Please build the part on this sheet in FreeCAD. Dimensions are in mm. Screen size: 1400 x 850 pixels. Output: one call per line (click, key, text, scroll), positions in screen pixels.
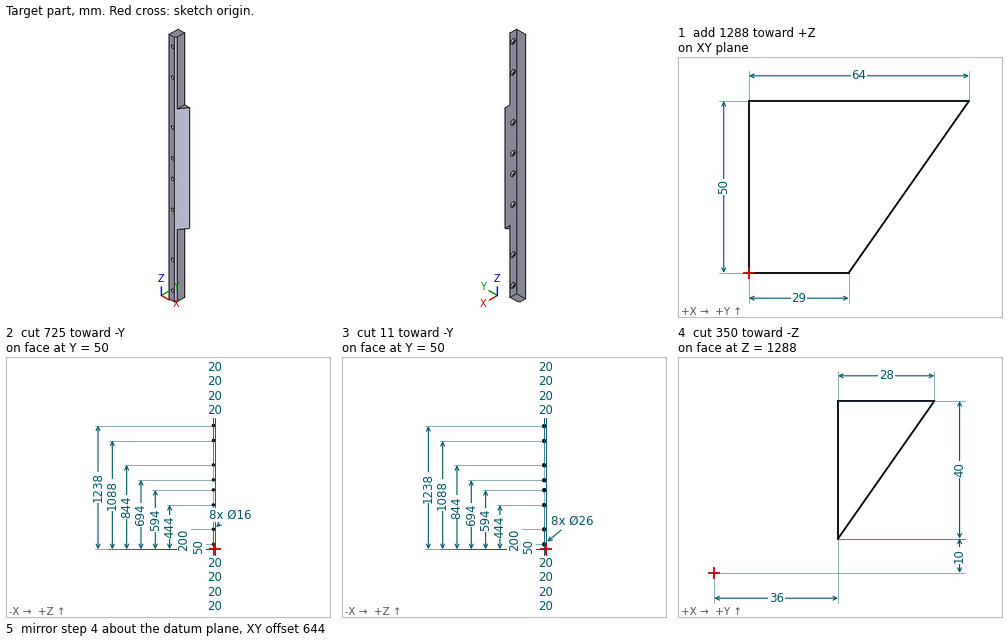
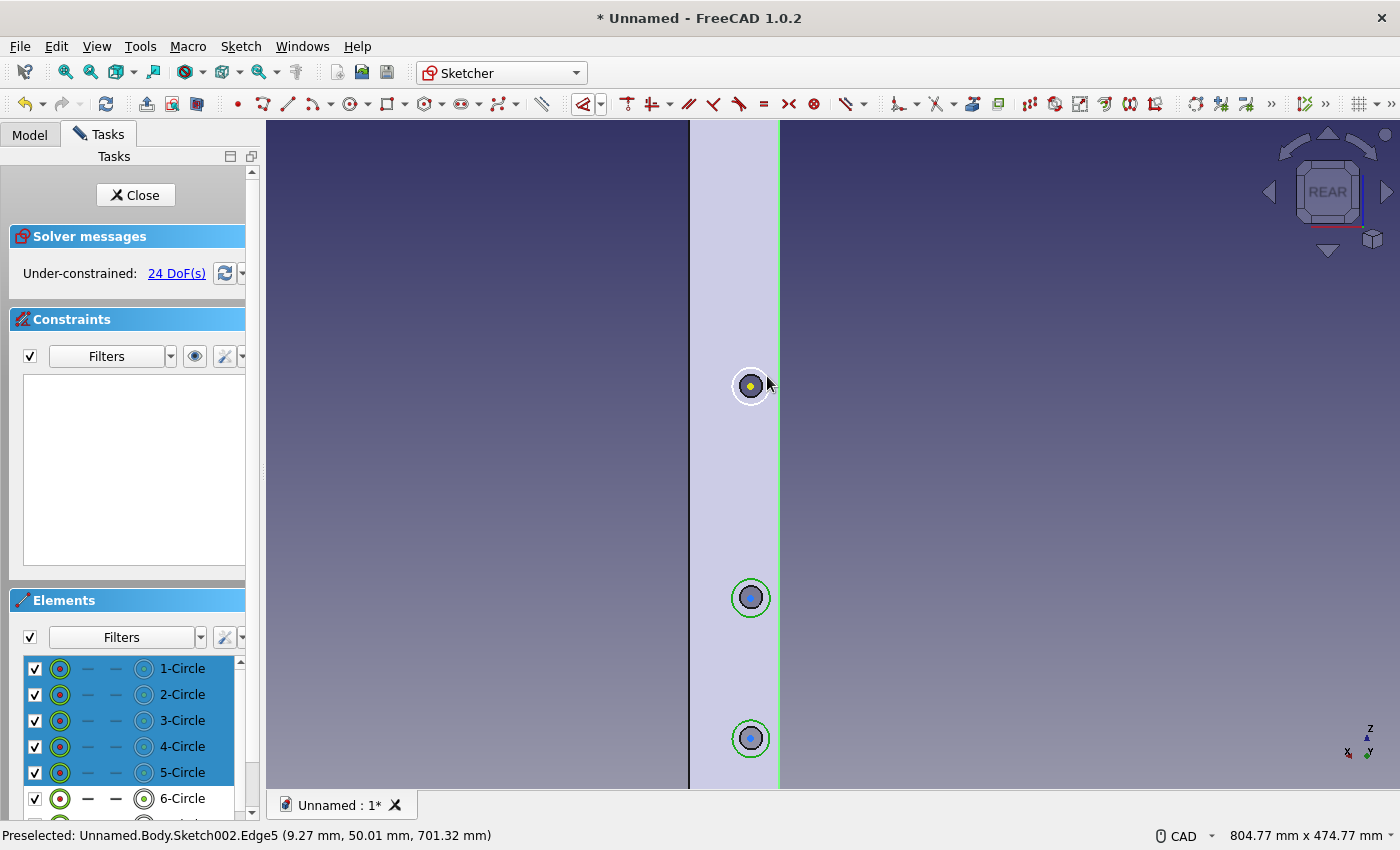
click(764, 373)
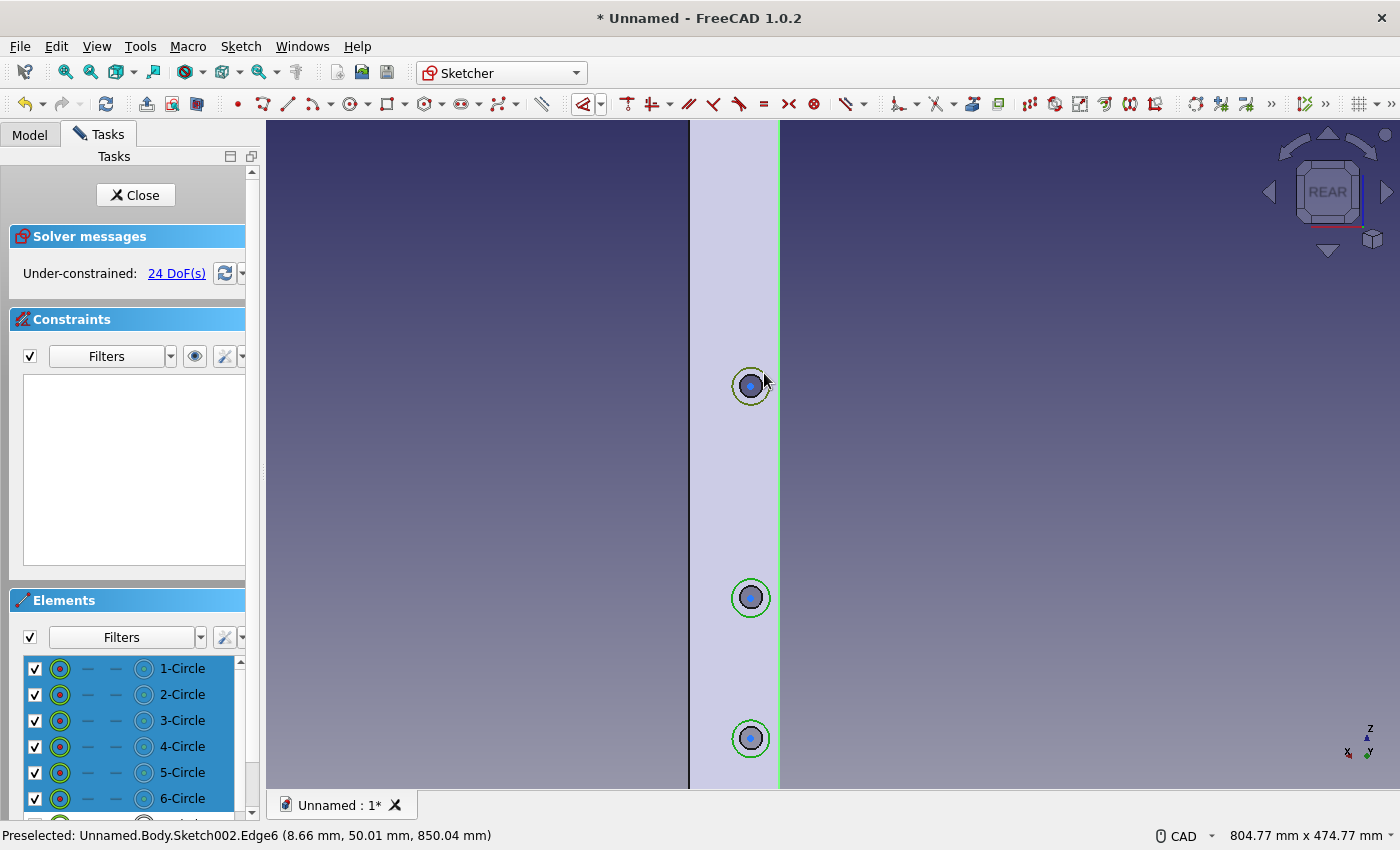
scroll(767, 376, down, 7)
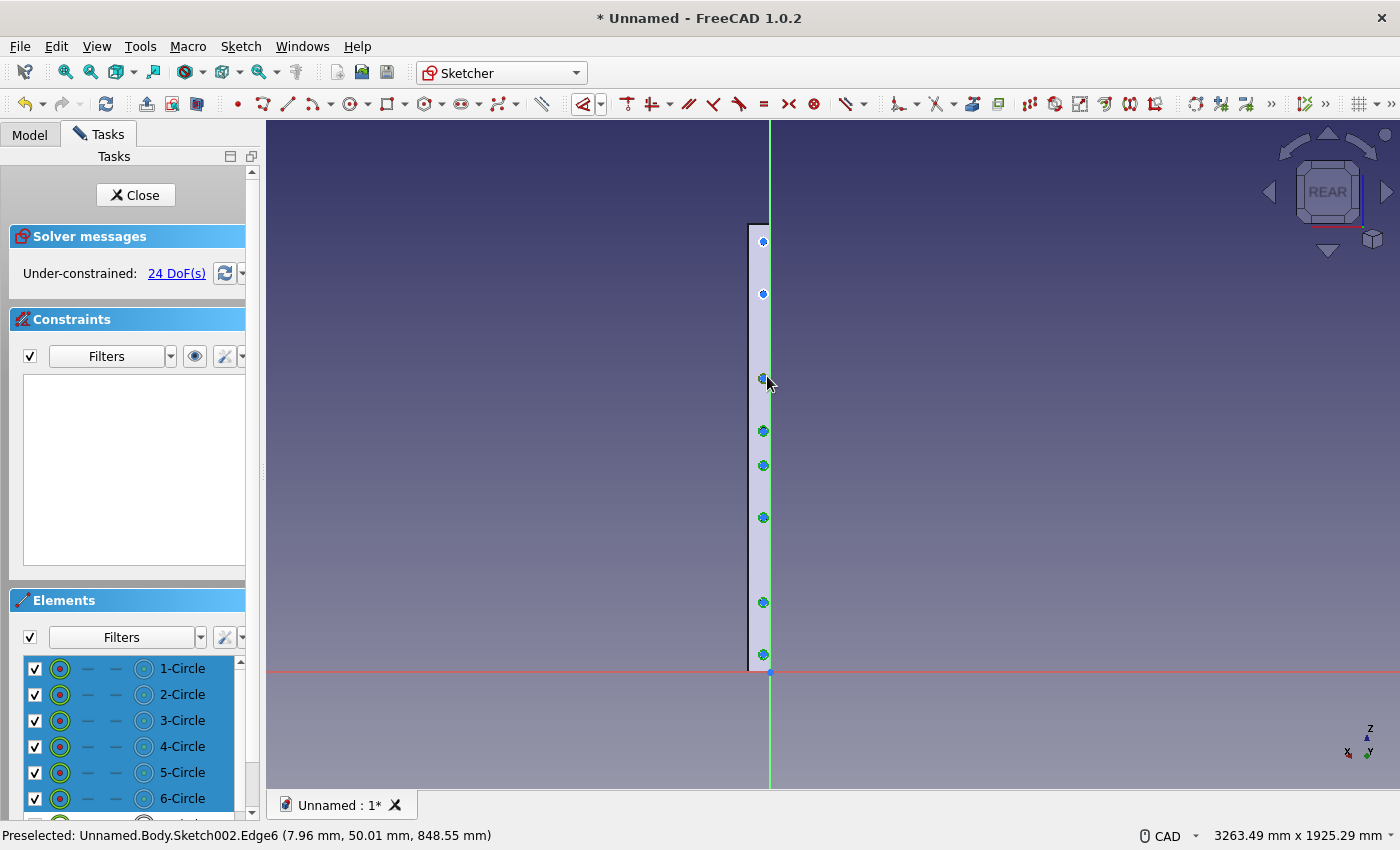
scroll(767, 291, up, 7)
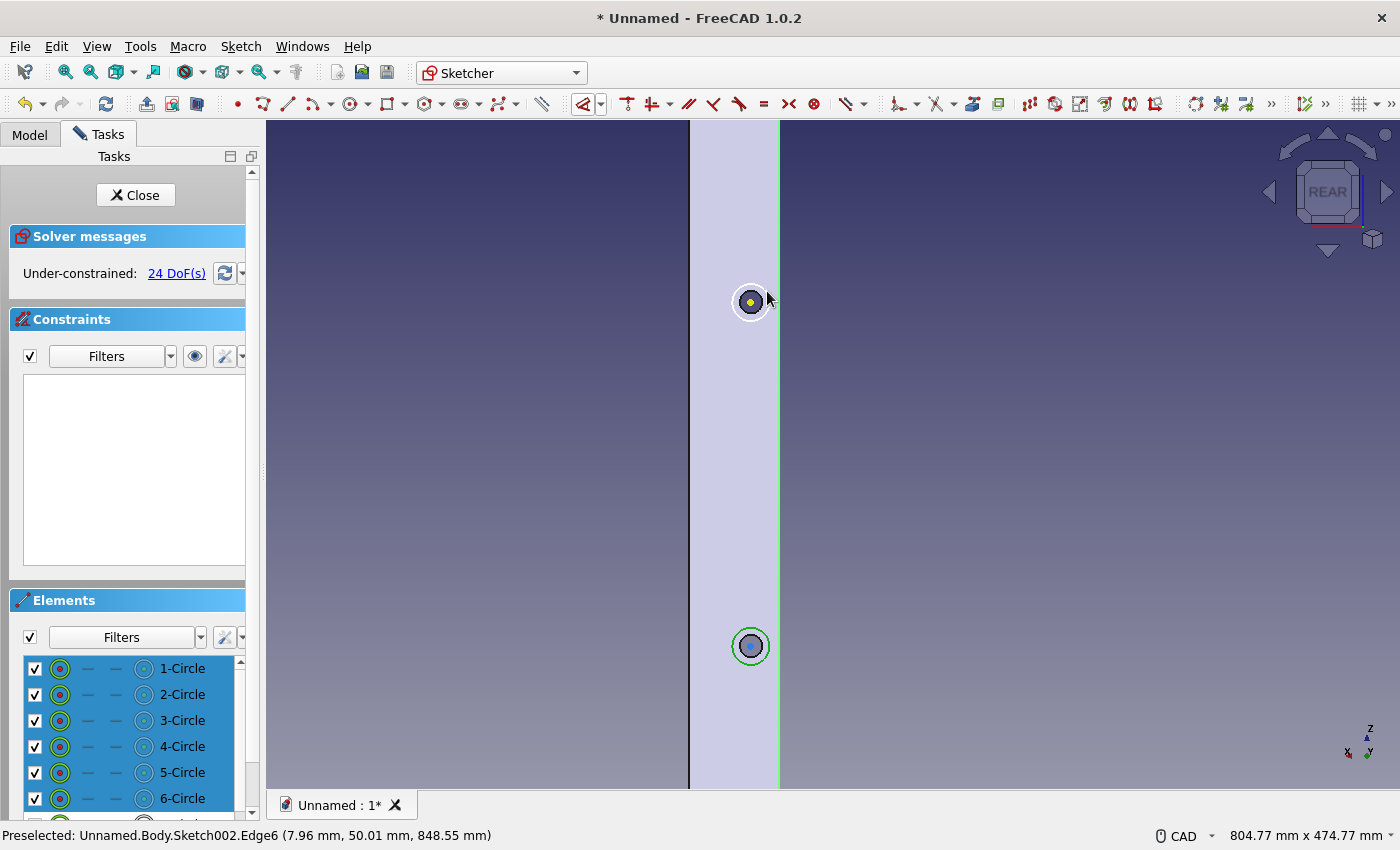
click(764, 289)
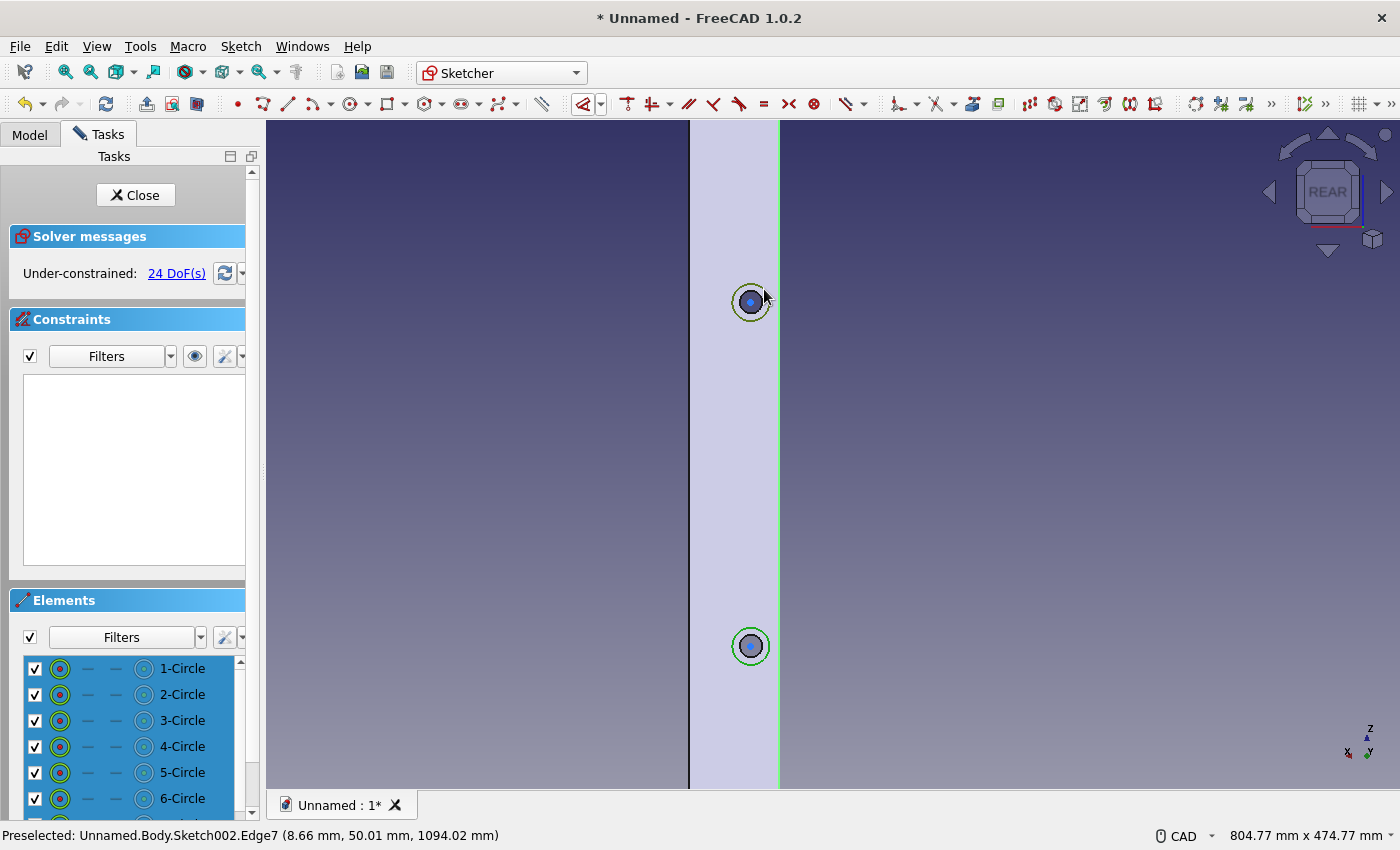
scroll(767, 291, down, 7)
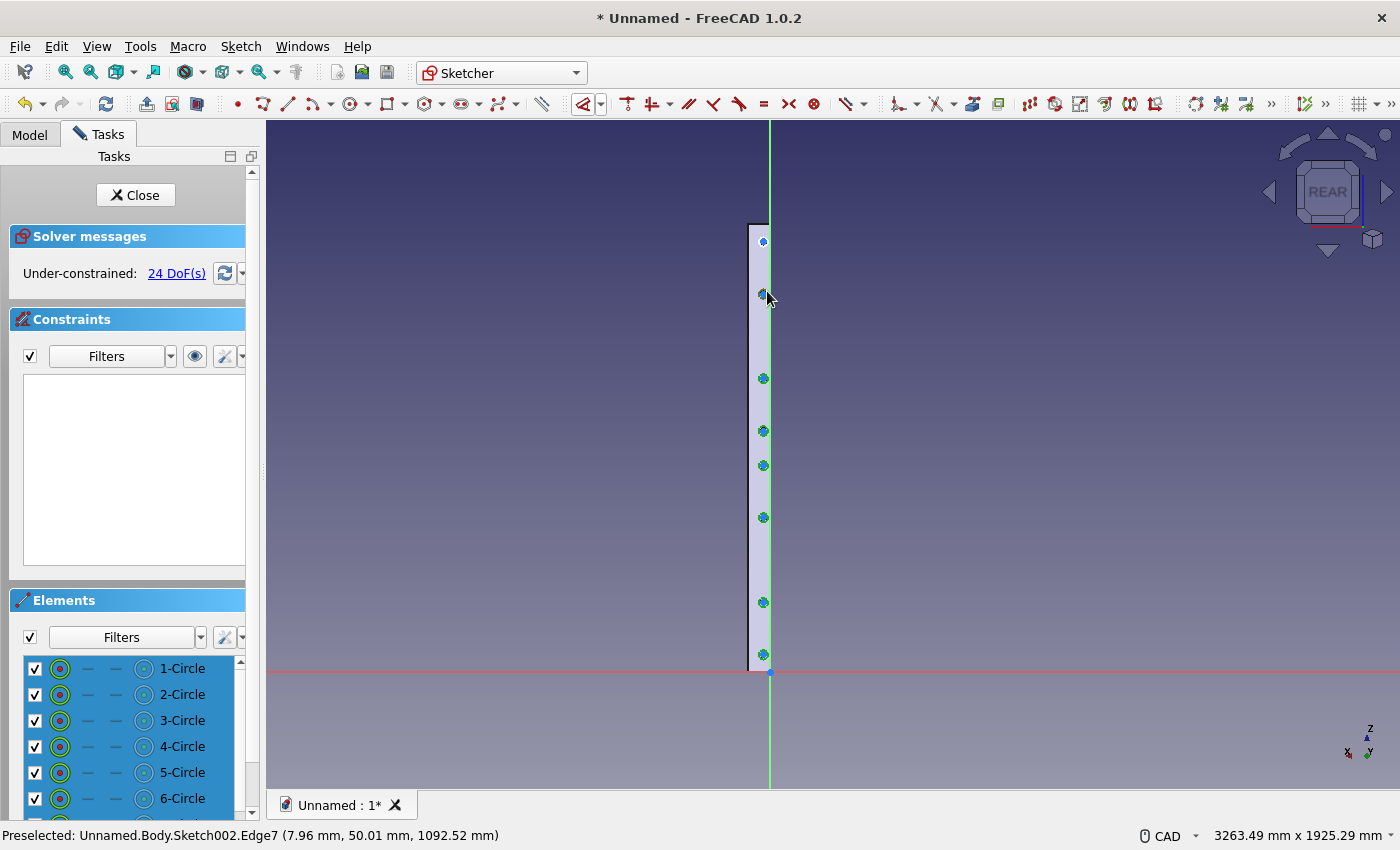
scroll(767, 239, up, 7)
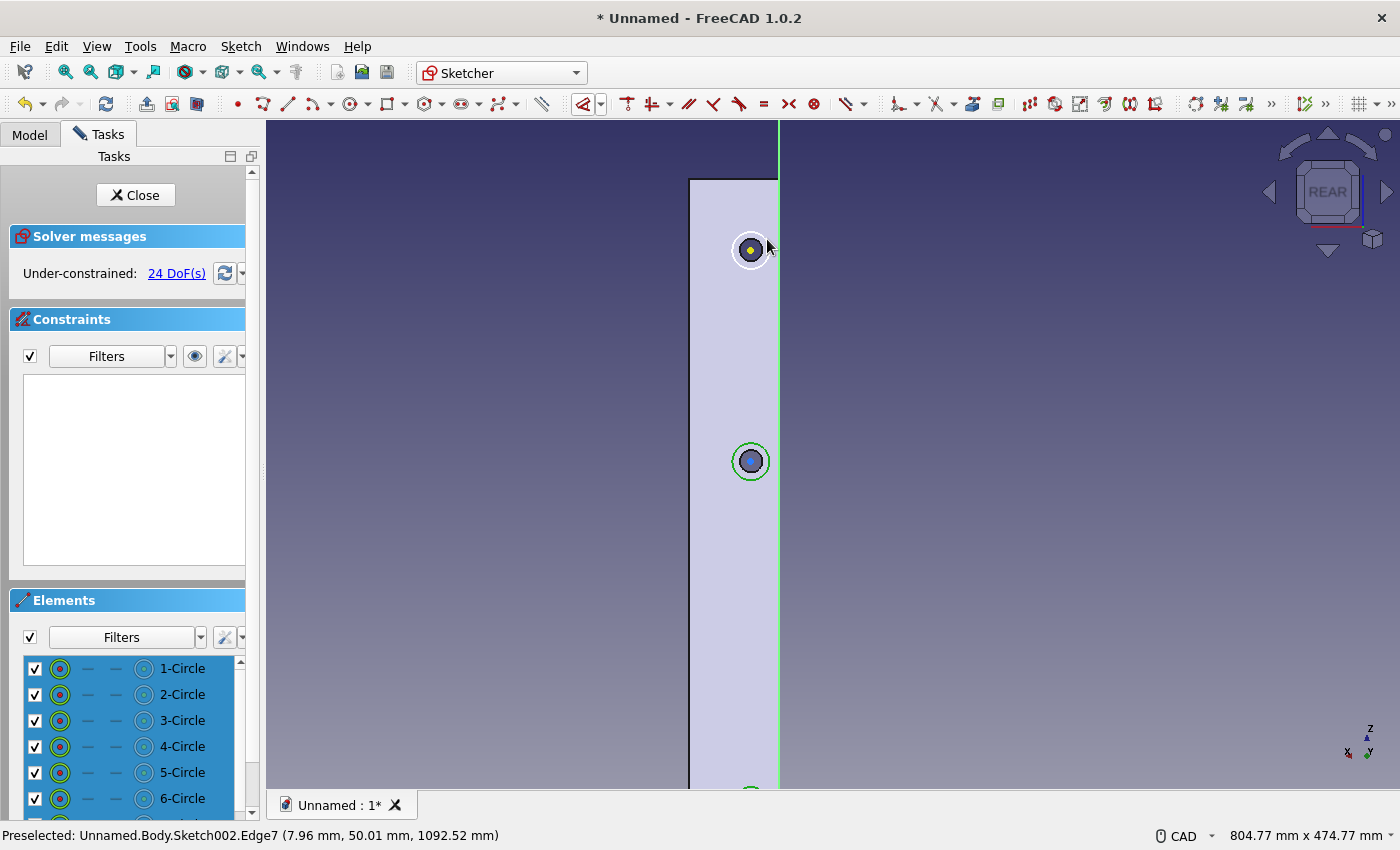
click(764, 237)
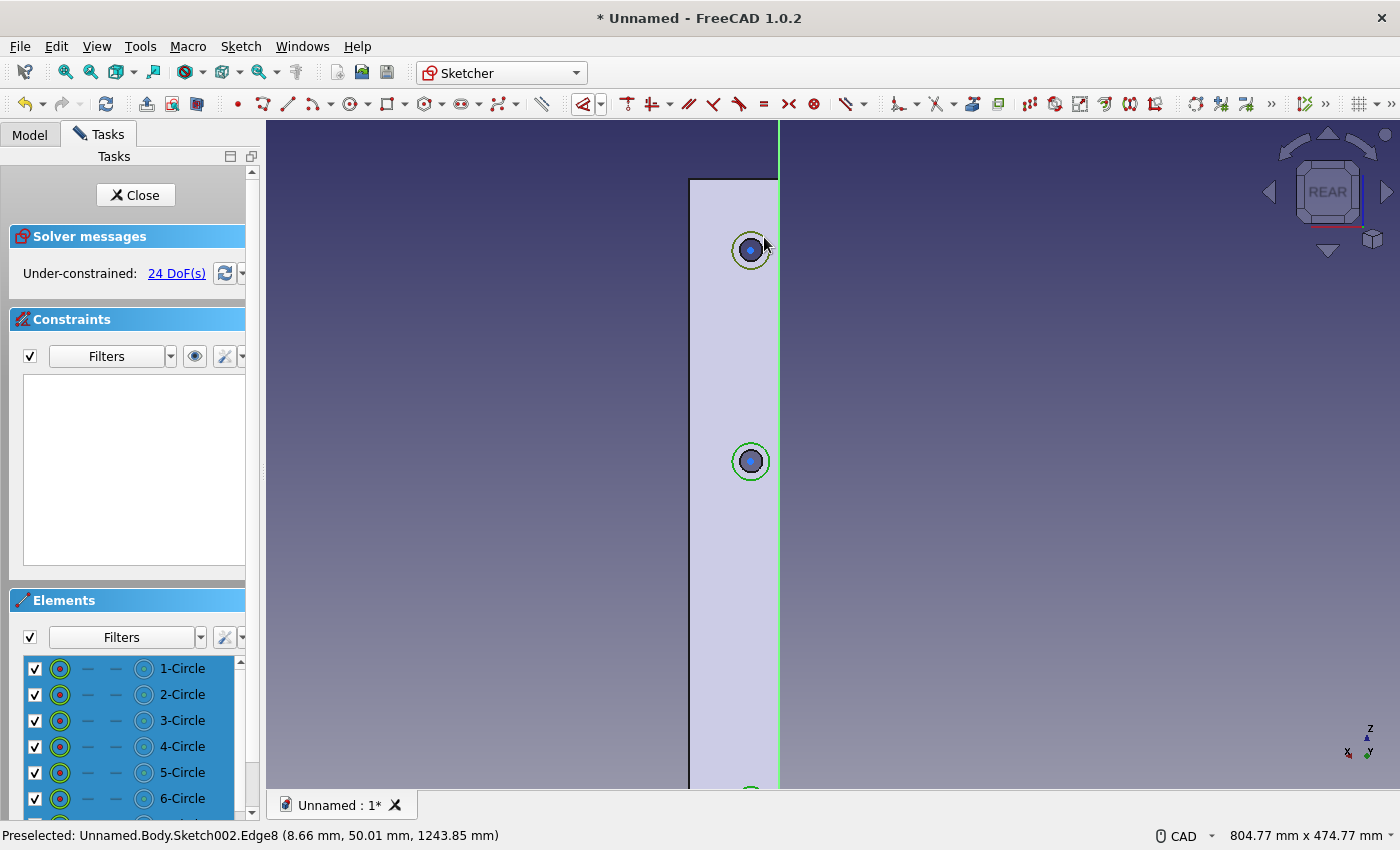
click(764, 104)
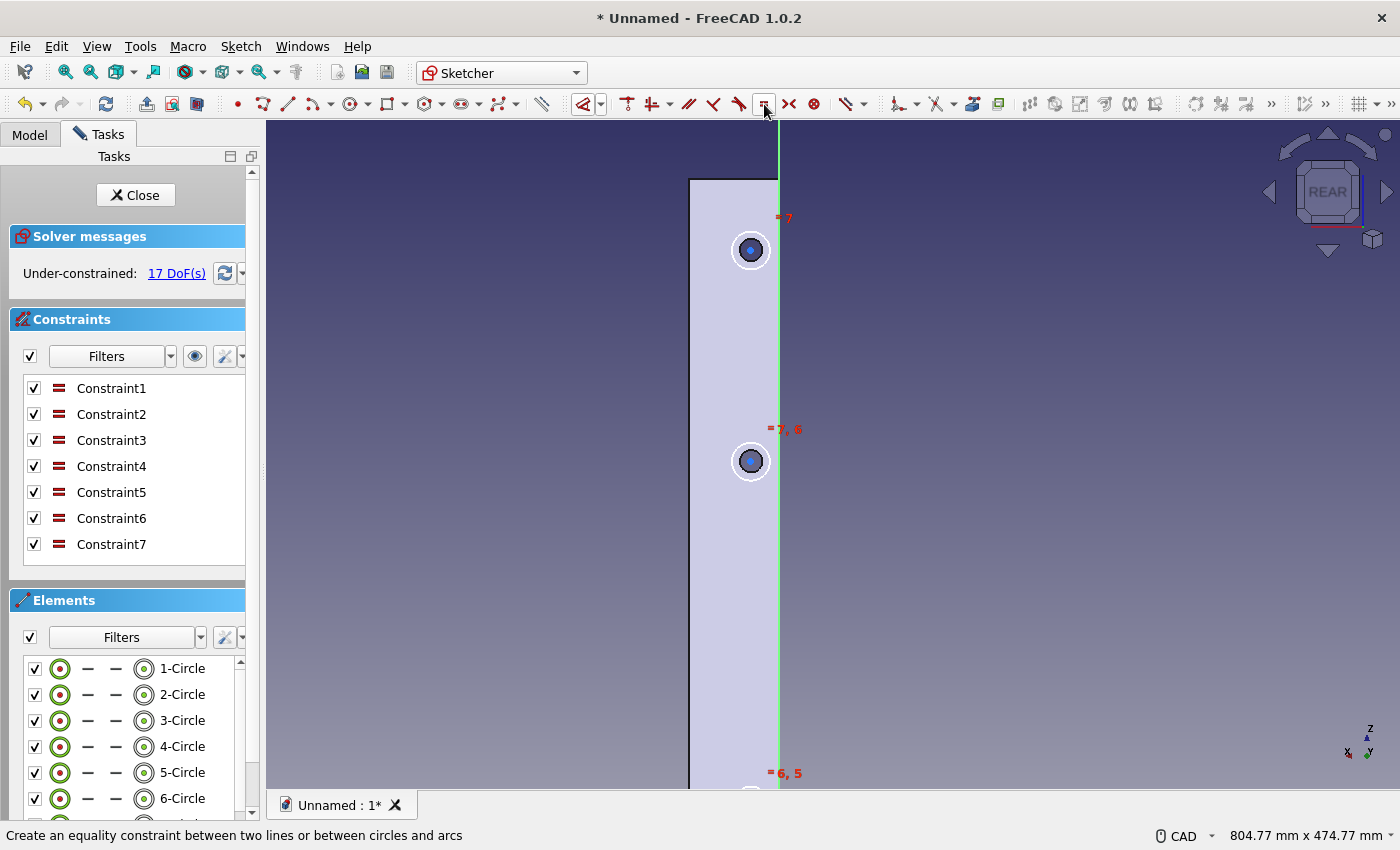
scroll(767, 239, down, 7)